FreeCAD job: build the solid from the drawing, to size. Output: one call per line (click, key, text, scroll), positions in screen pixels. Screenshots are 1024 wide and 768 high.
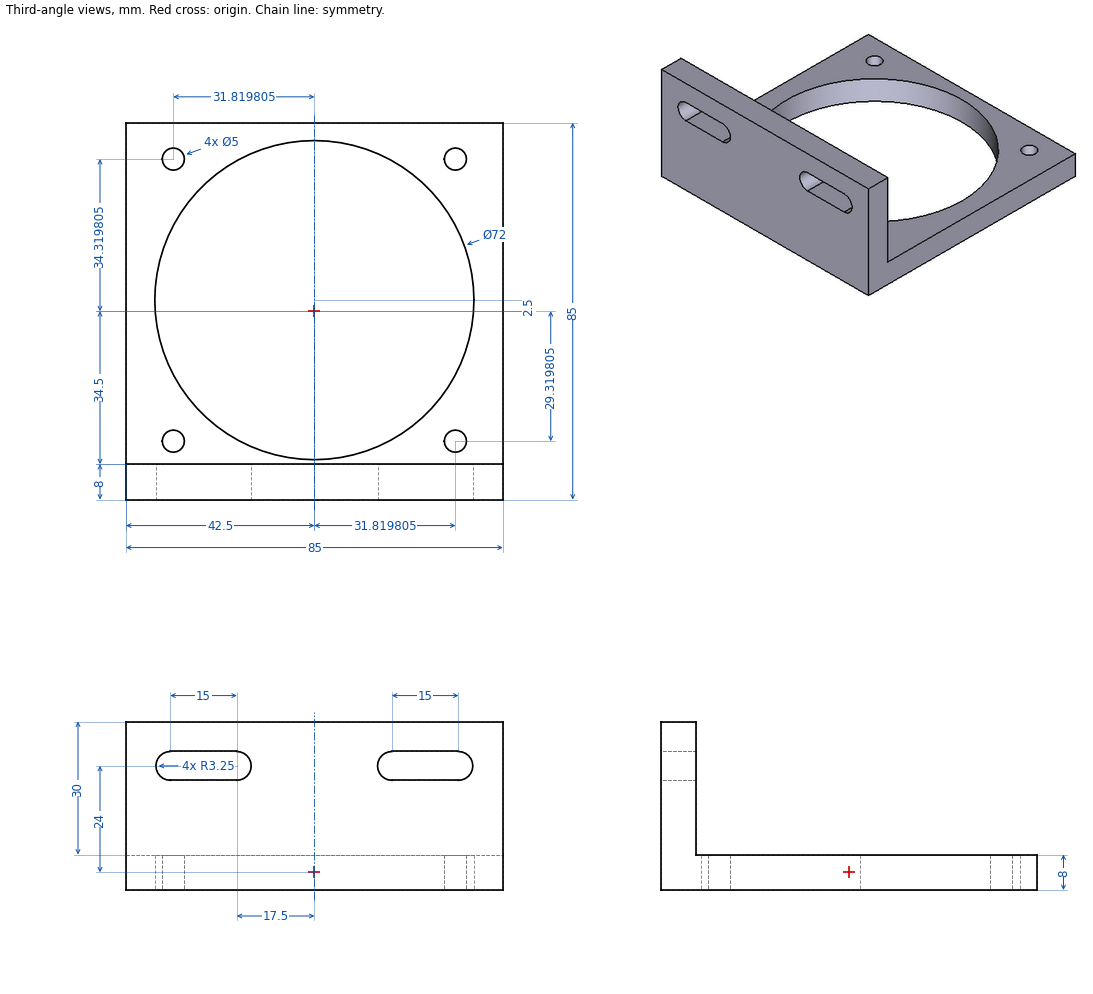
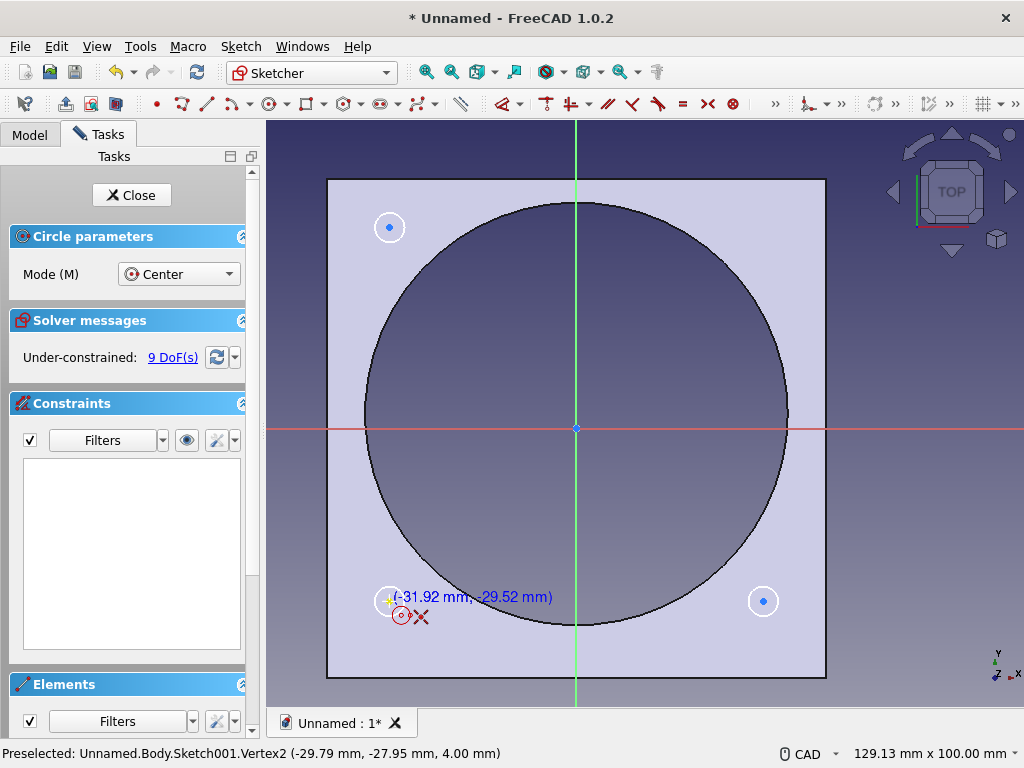
scroll(763, 227, up, 3)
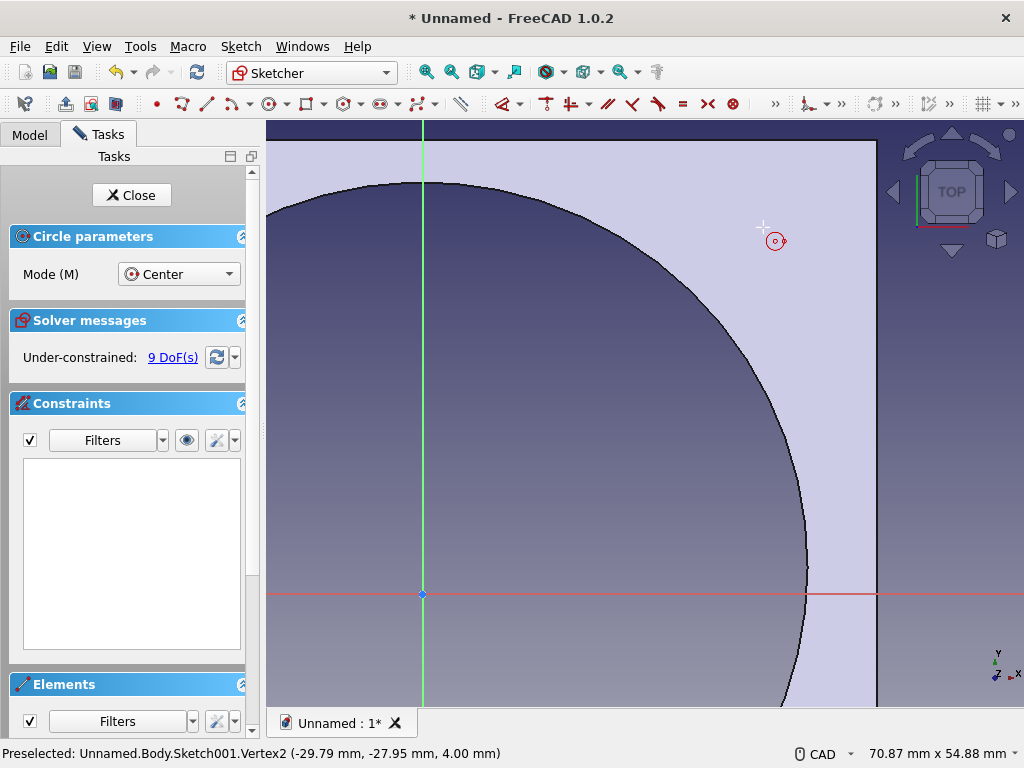
click(763, 227)
click(782, 208)
key(Escape)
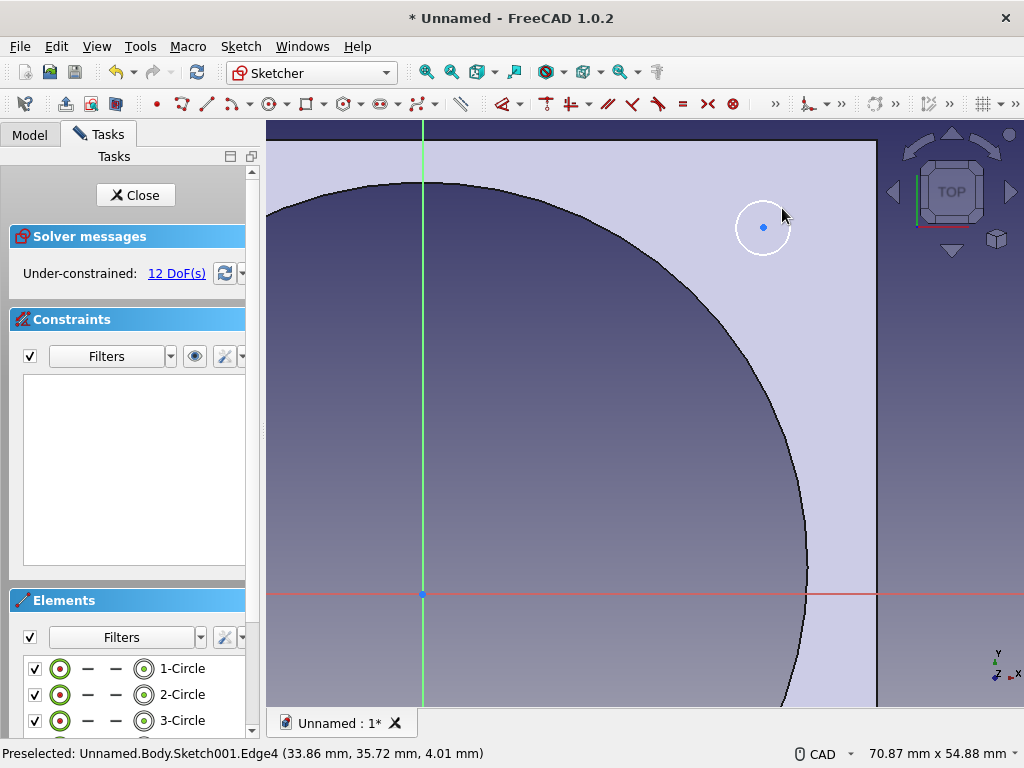
scroll(764, 226, down, 3)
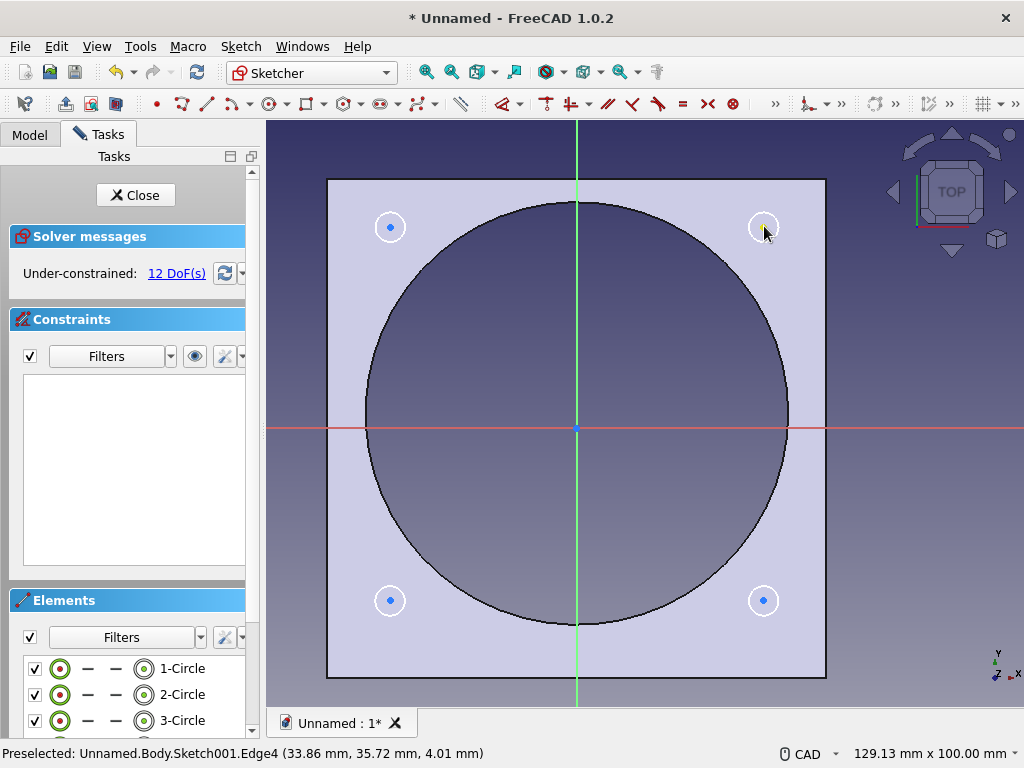
click(401, 217)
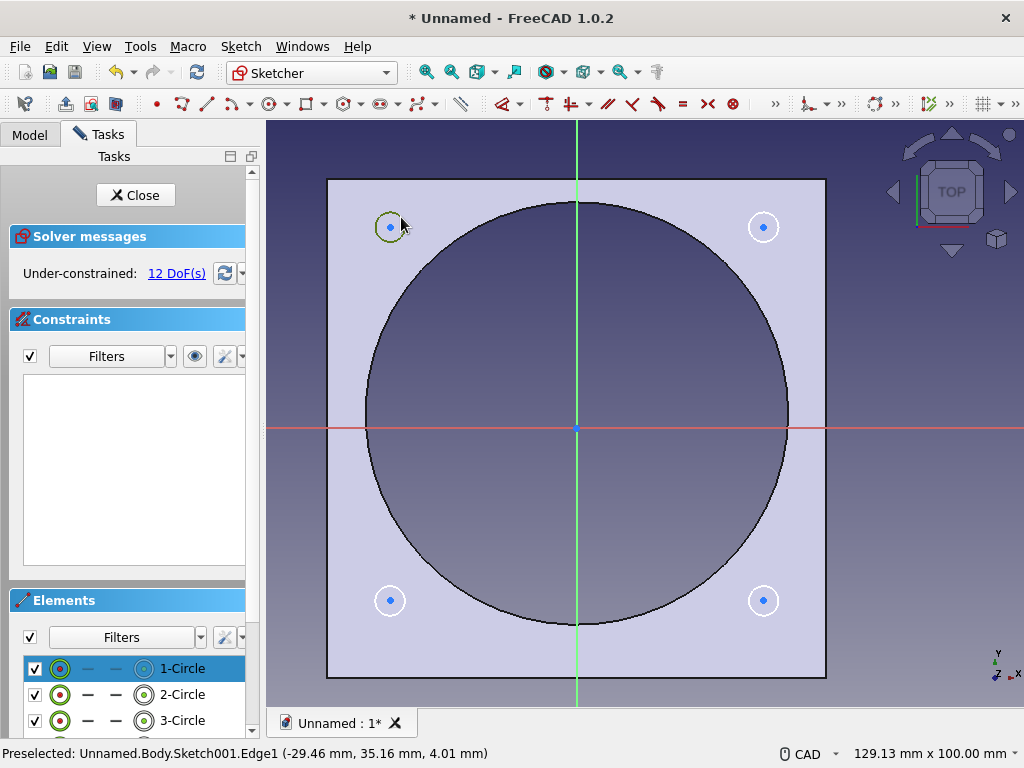
click(774, 590)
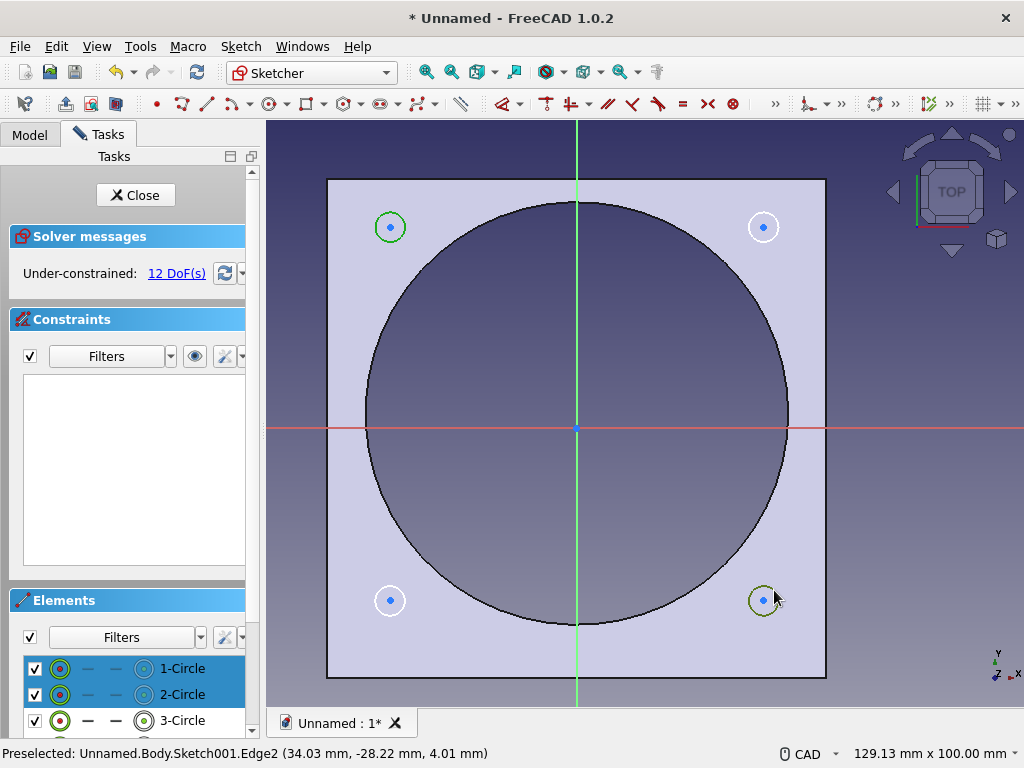
click(400, 590)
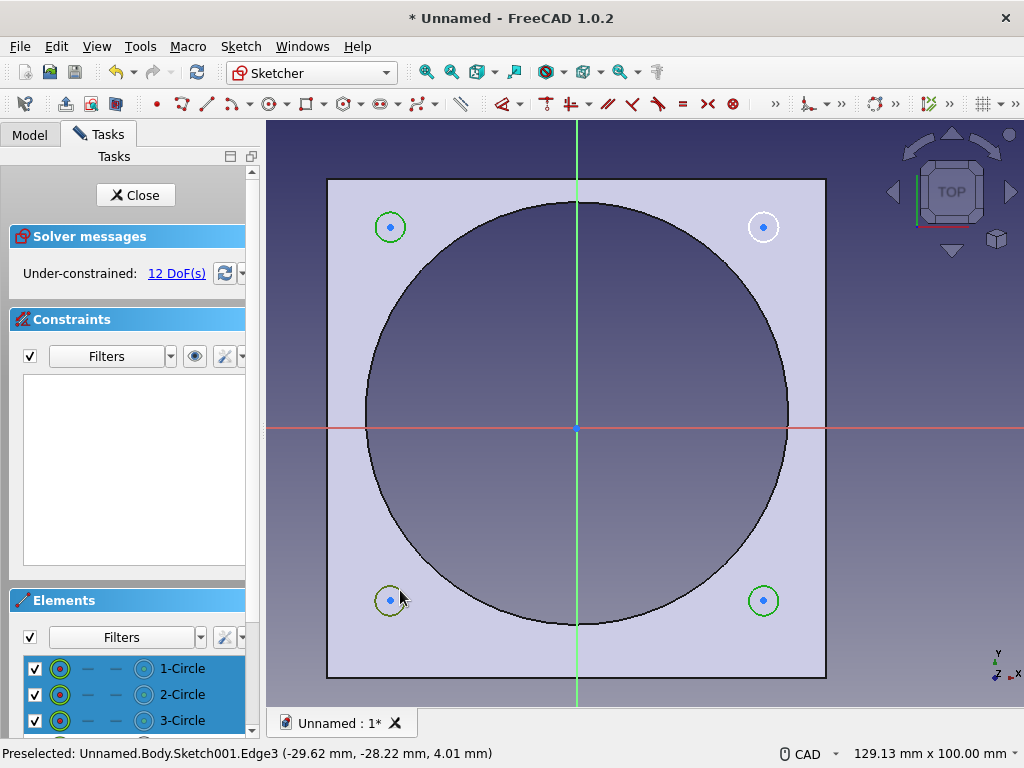
click(774, 217)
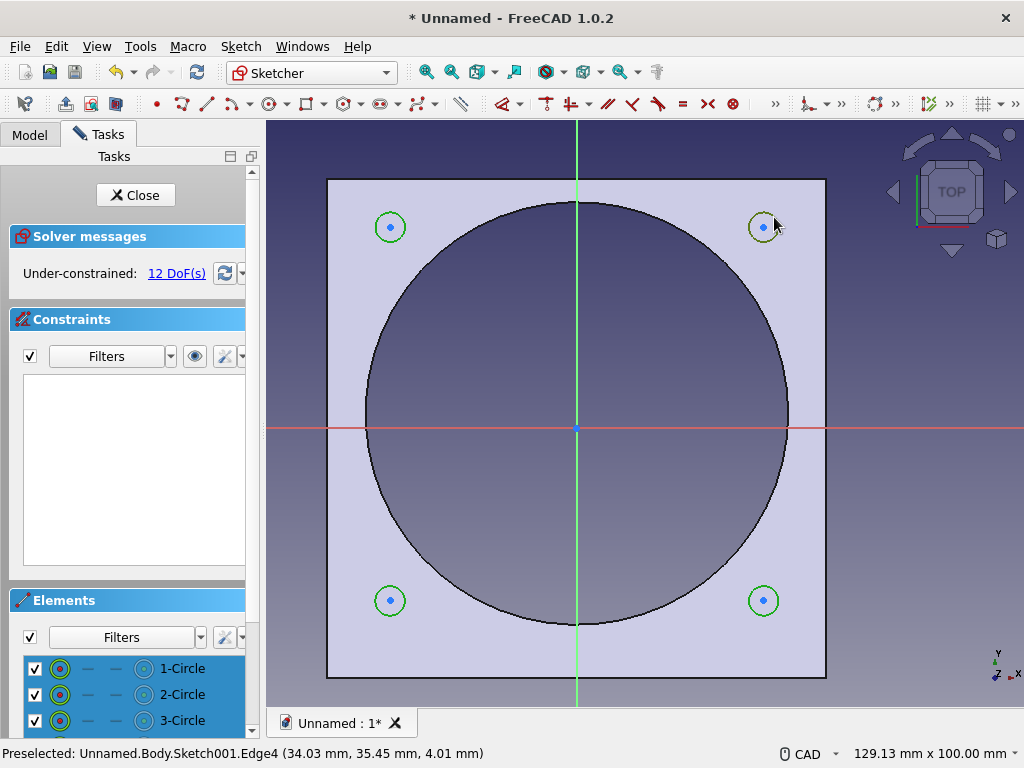
key(e)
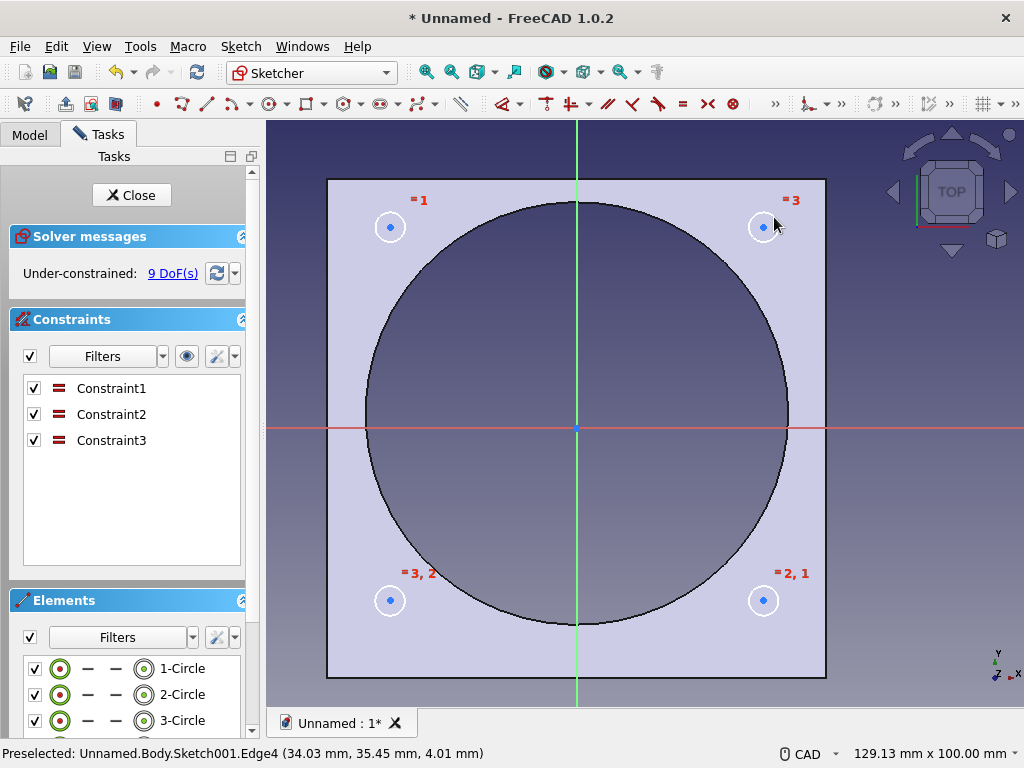
click(764, 601)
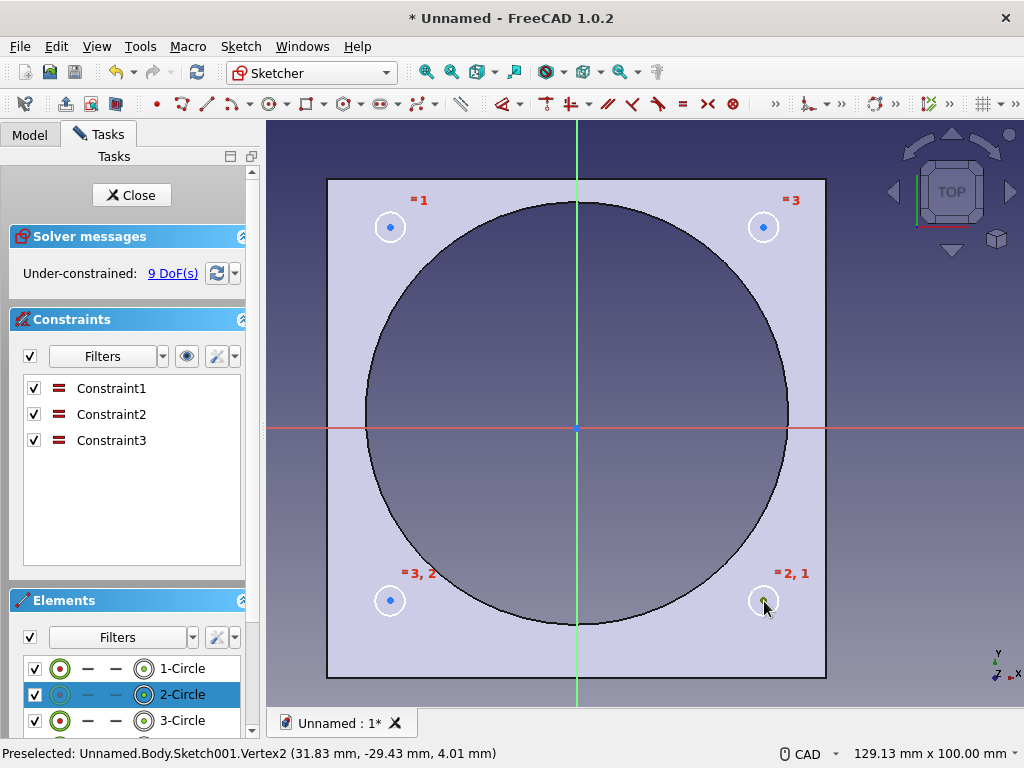
click(390, 601)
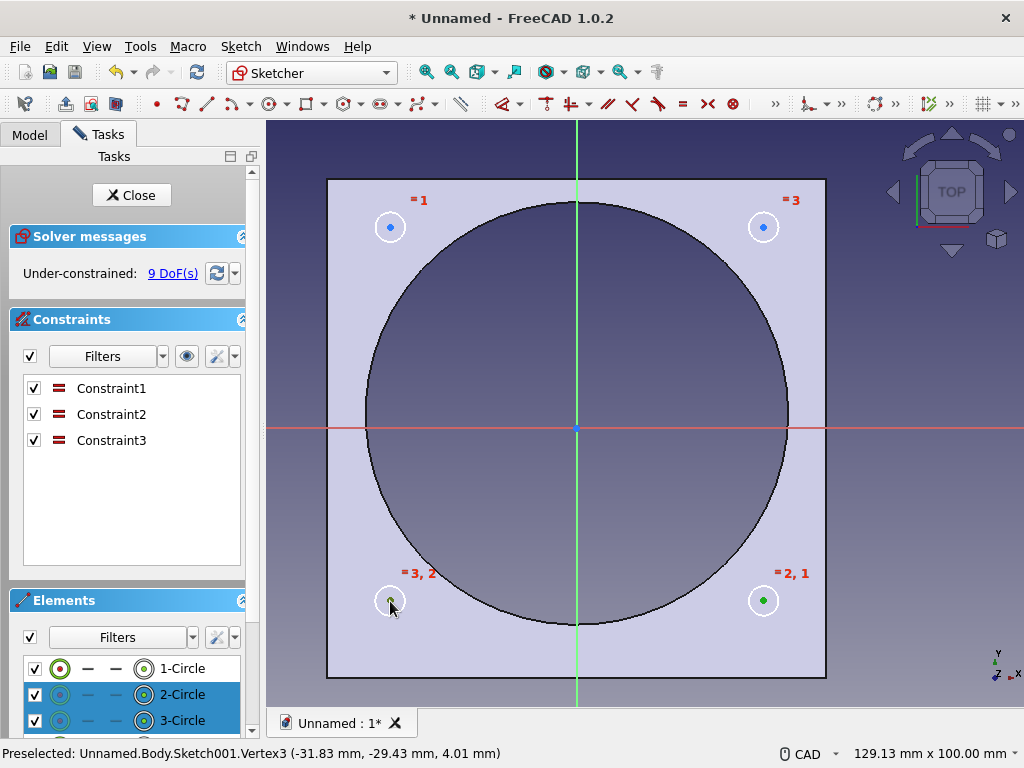
click(577, 641)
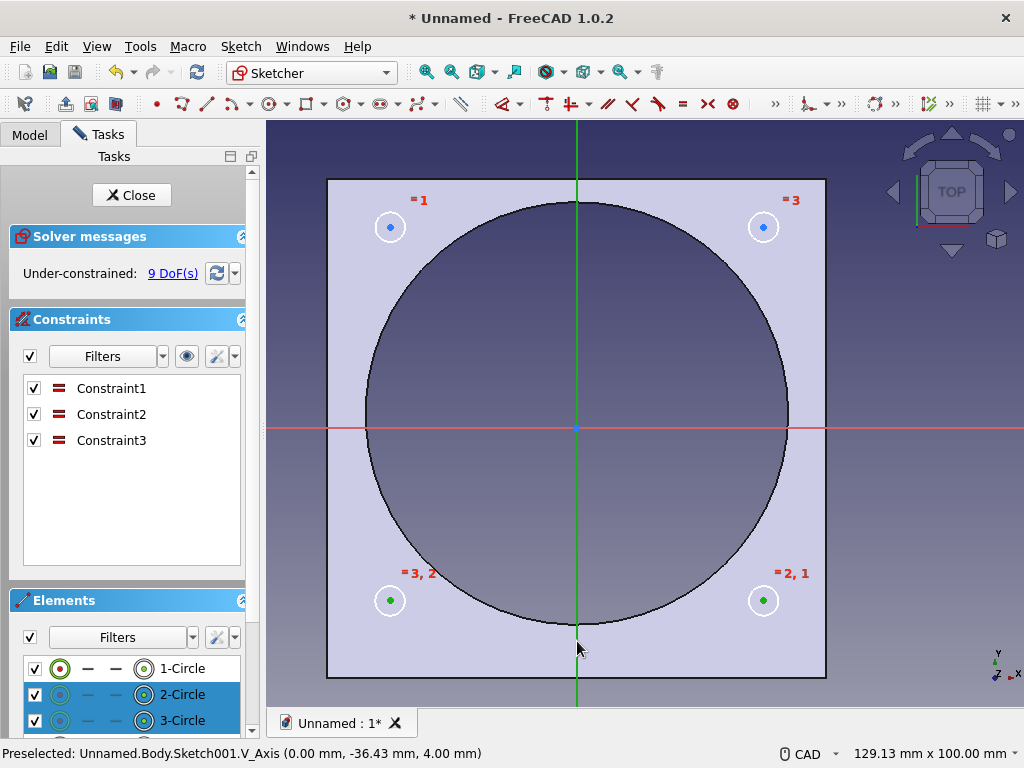
click(708, 104)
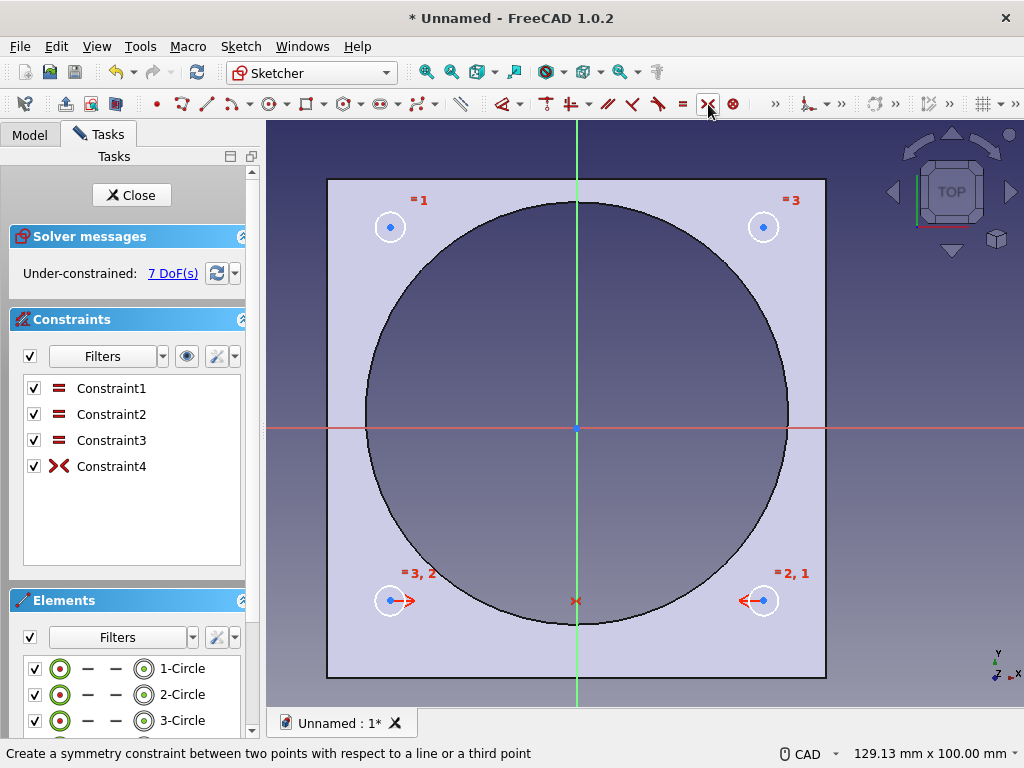
click(390, 227)